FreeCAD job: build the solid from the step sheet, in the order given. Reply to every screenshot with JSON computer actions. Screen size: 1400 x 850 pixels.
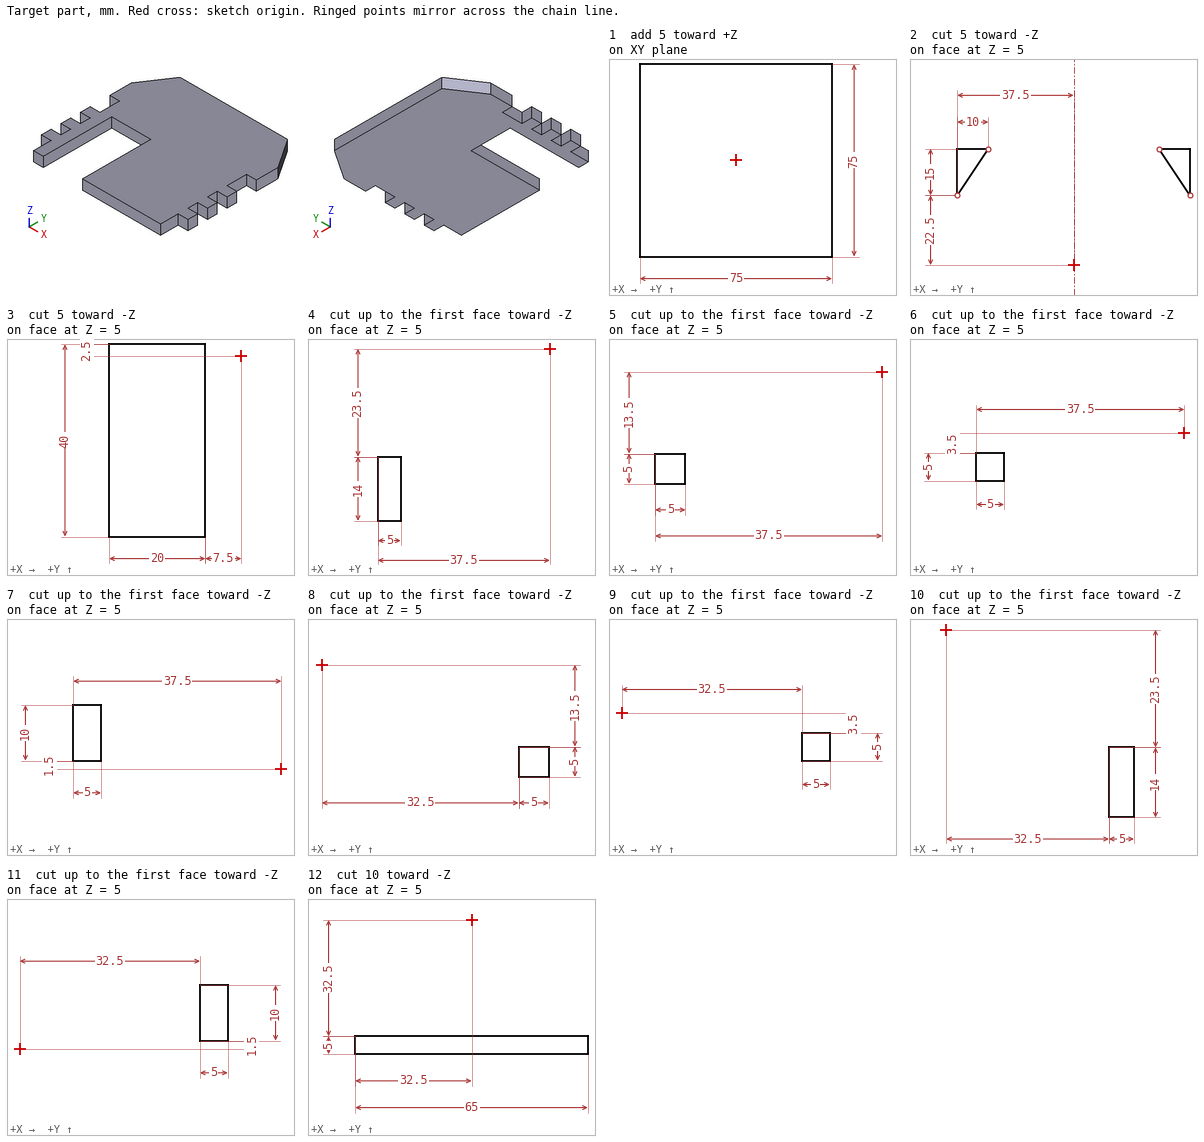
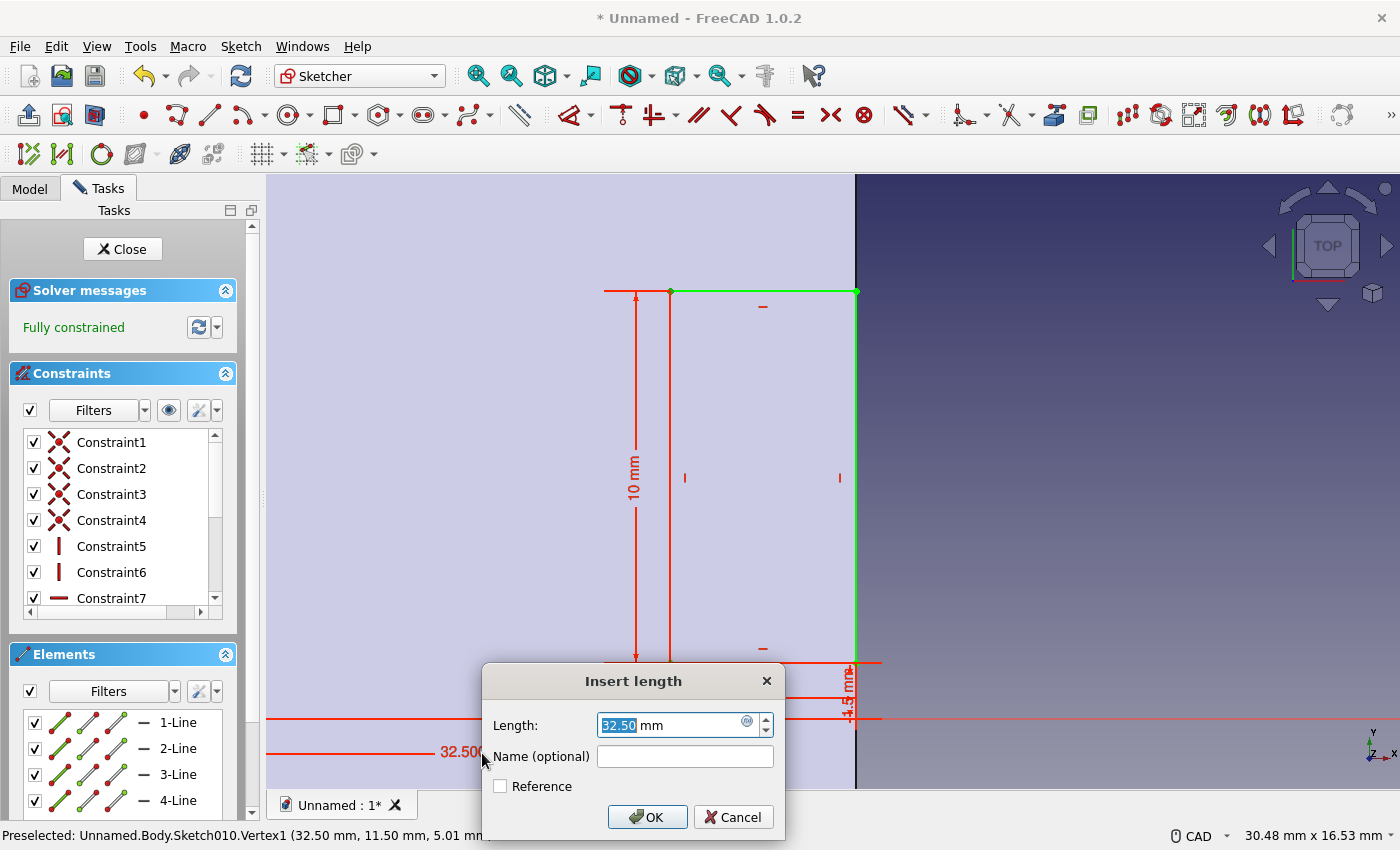
{"action": "type", "text": "32.5"}
{"action": "key", "text": "Return"}
{"action": "key", "text": "Escape"}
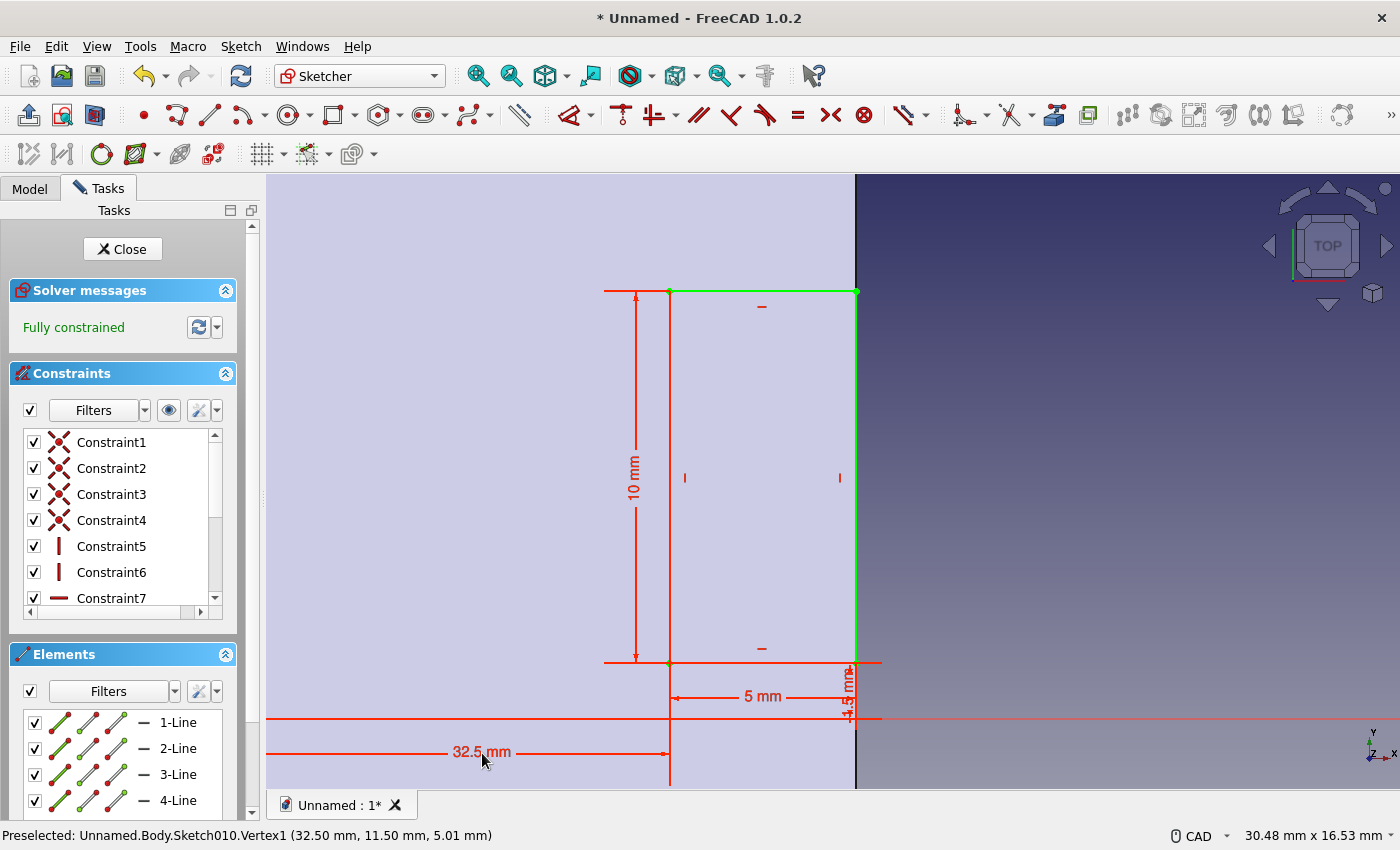
{"action": "left_click", "coordinate": [123, 249]}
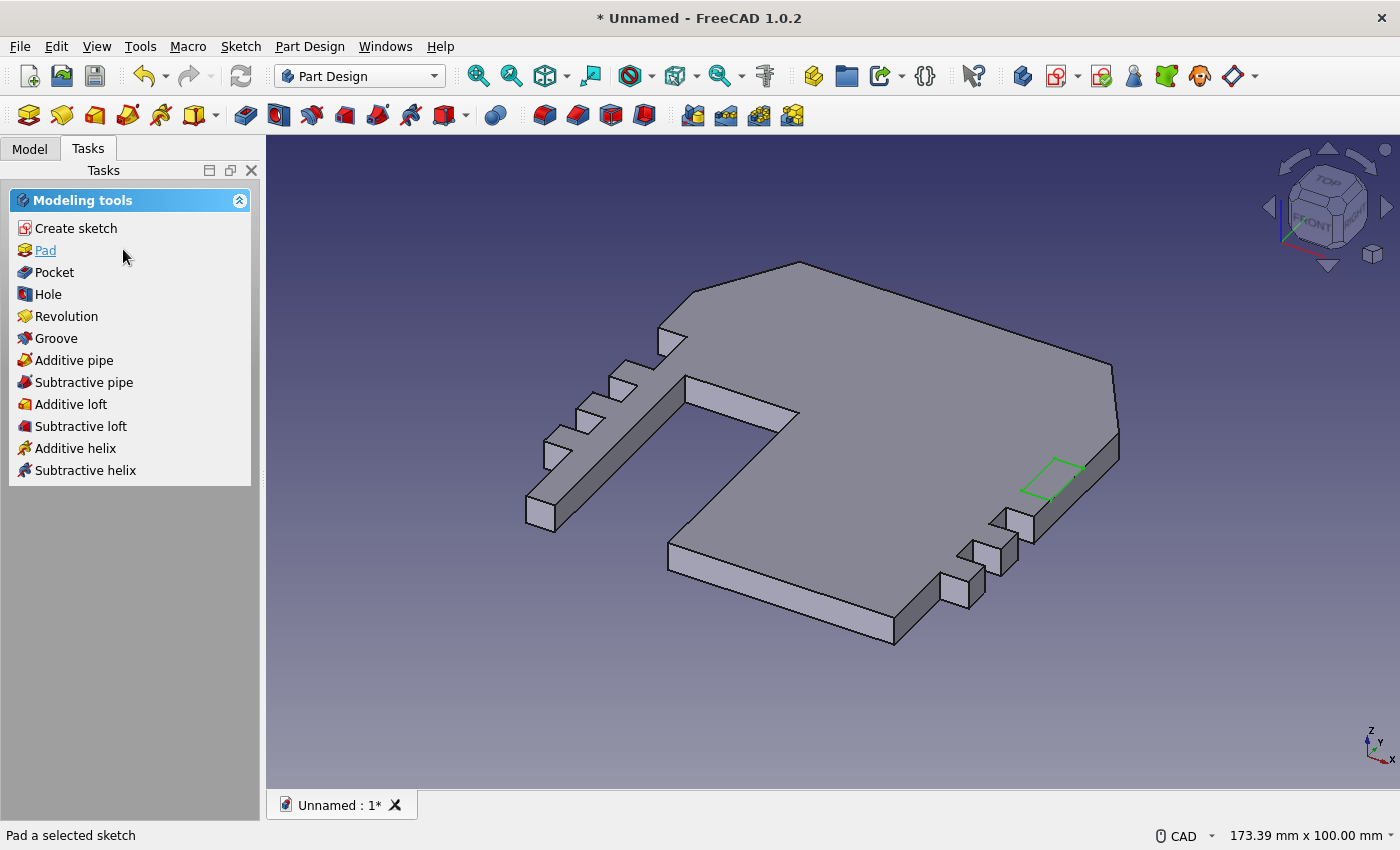
{"action": "left_click", "coordinate": [246, 116]}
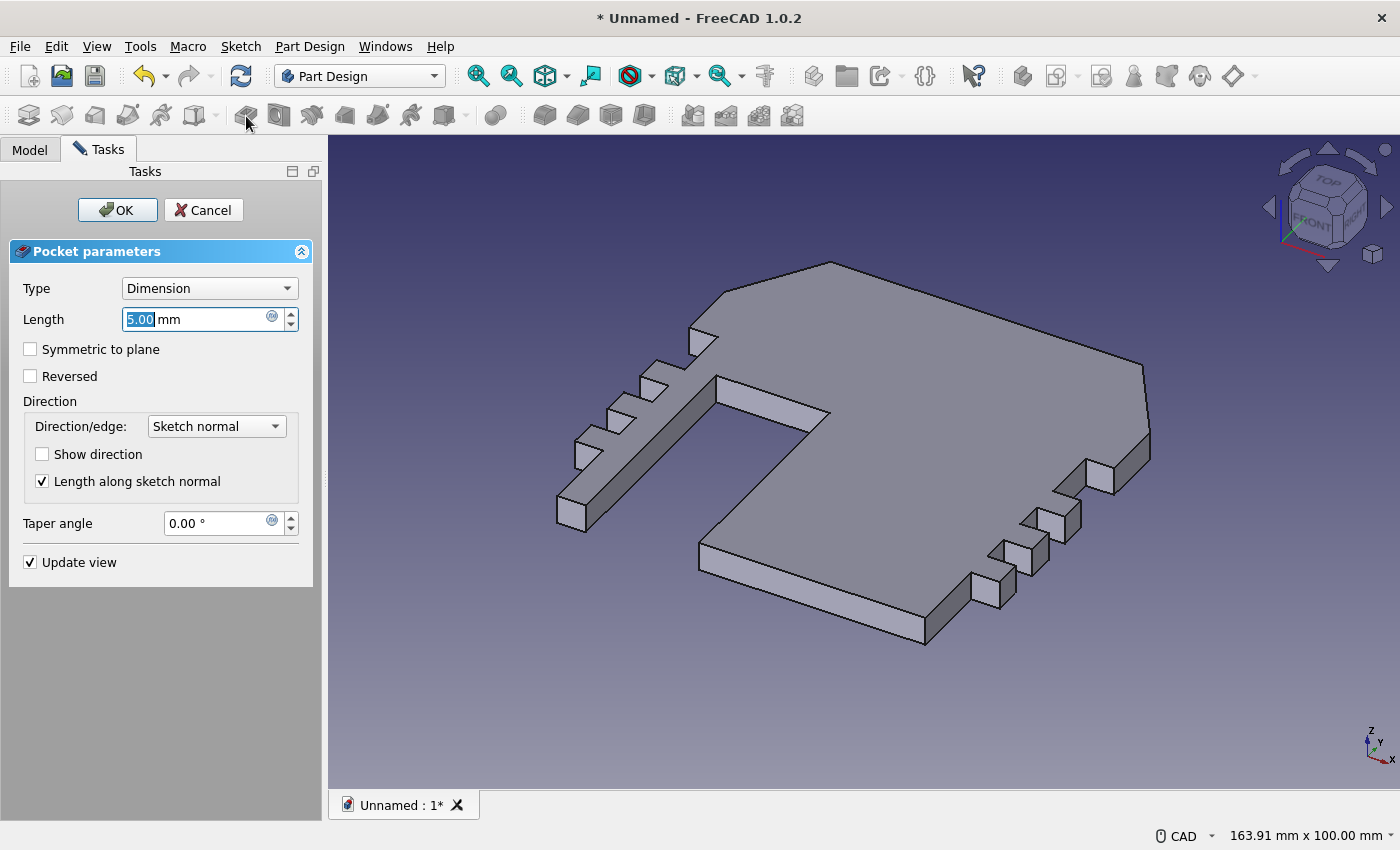
{"action": "left_click", "coordinate": [210, 288]}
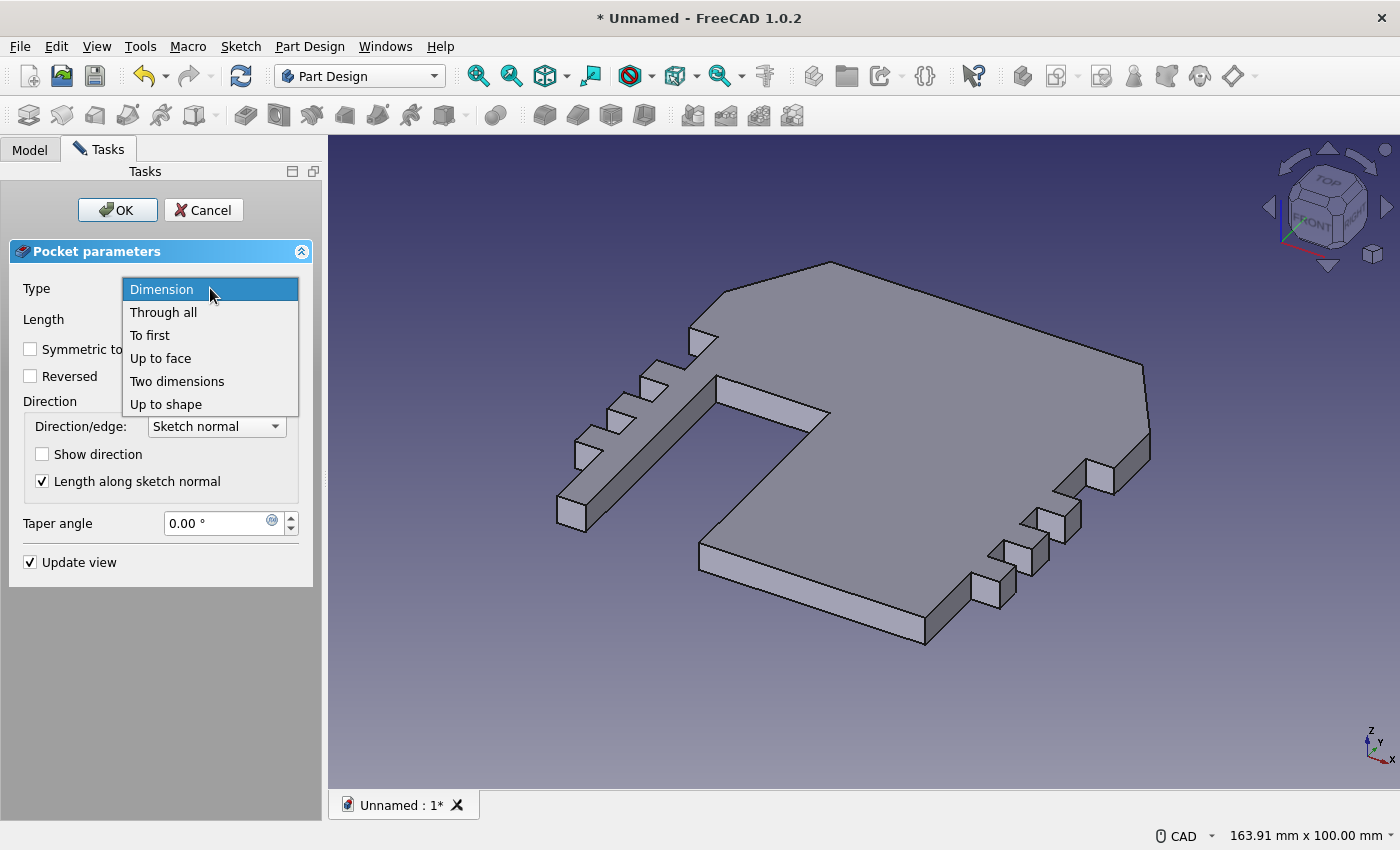
{"action": "left_click", "coordinate": [208, 336]}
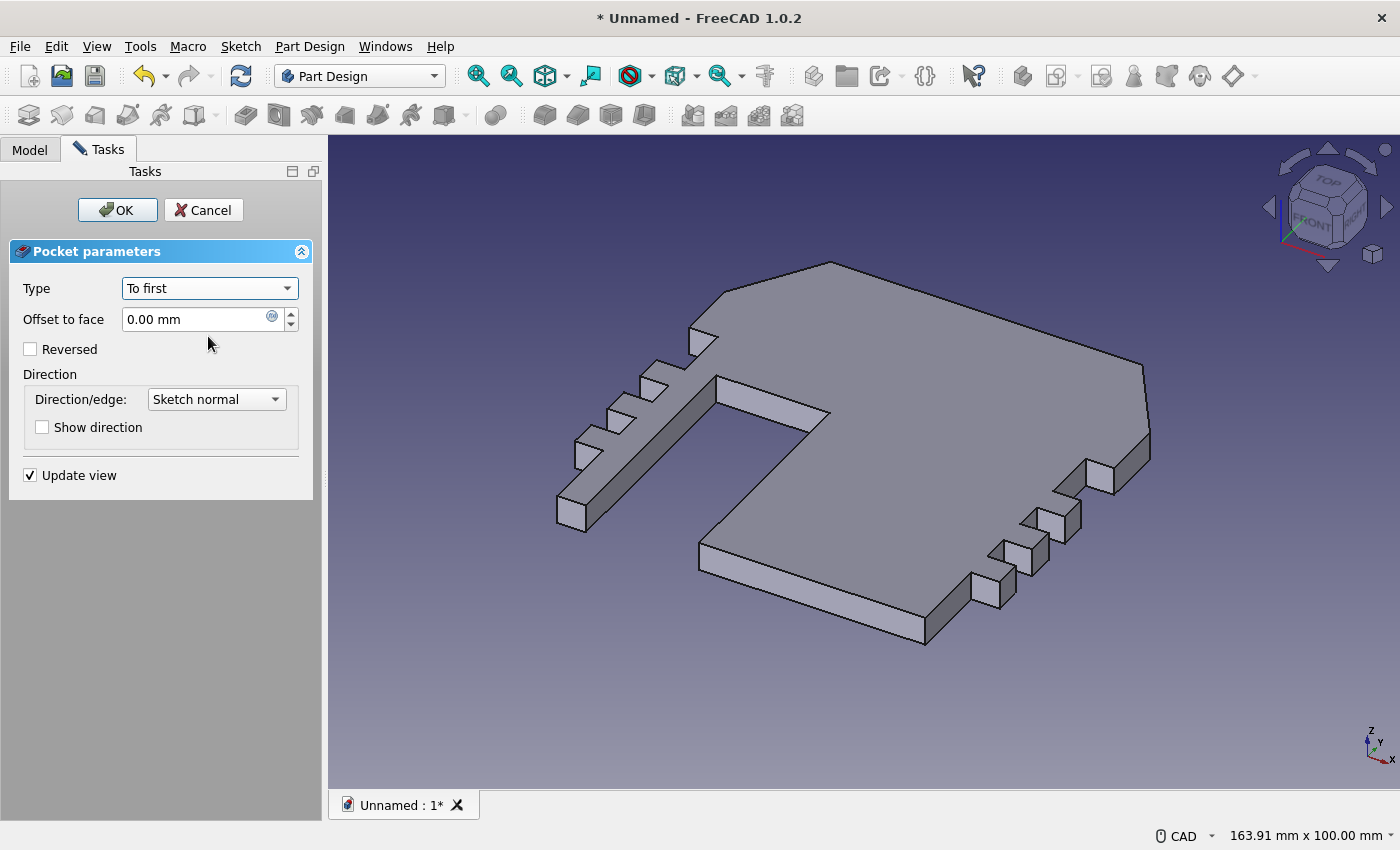
{"action": "left_click", "coordinate": [118, 210]}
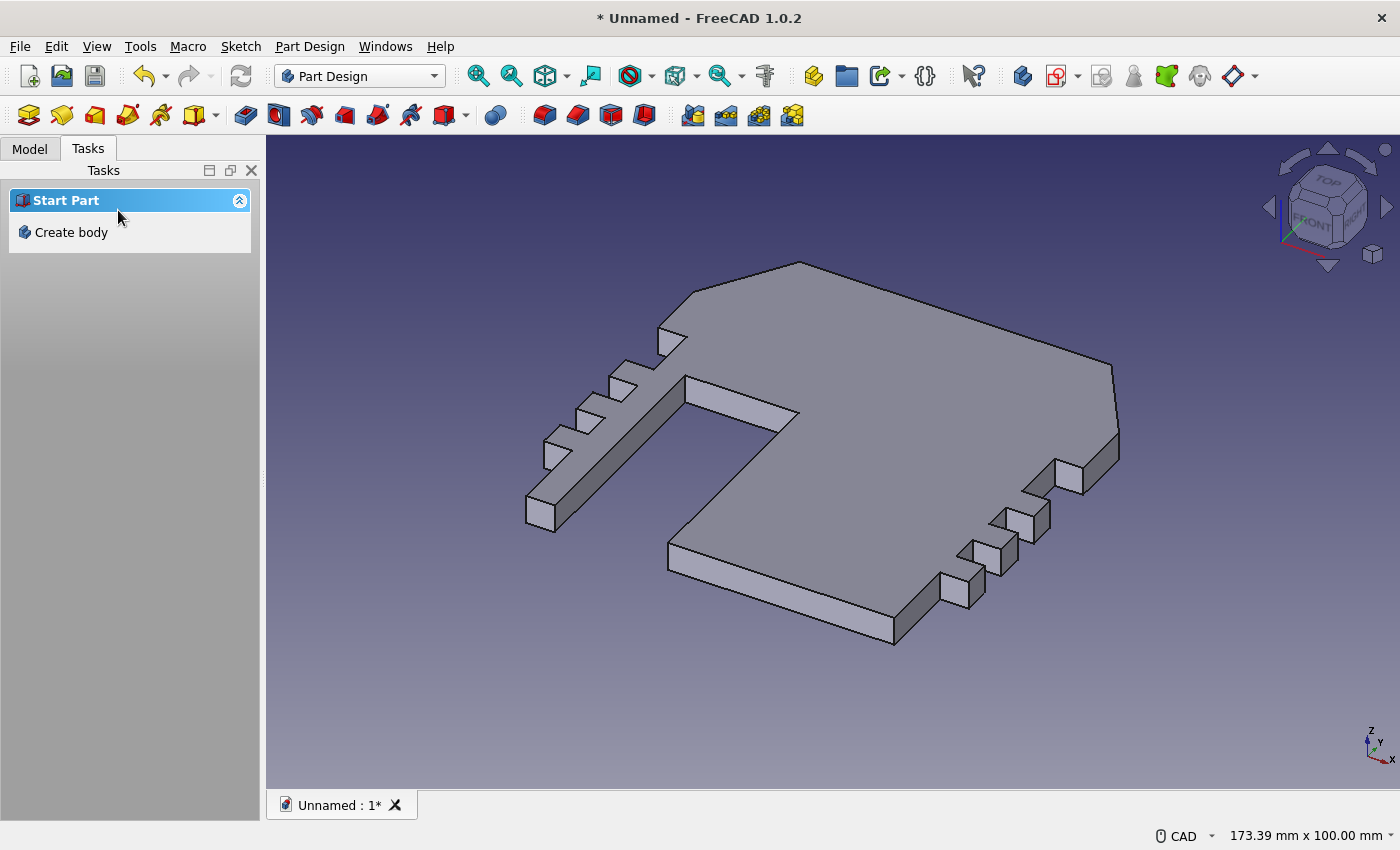
{"action": "left_click", "coordinate": [929, 420]}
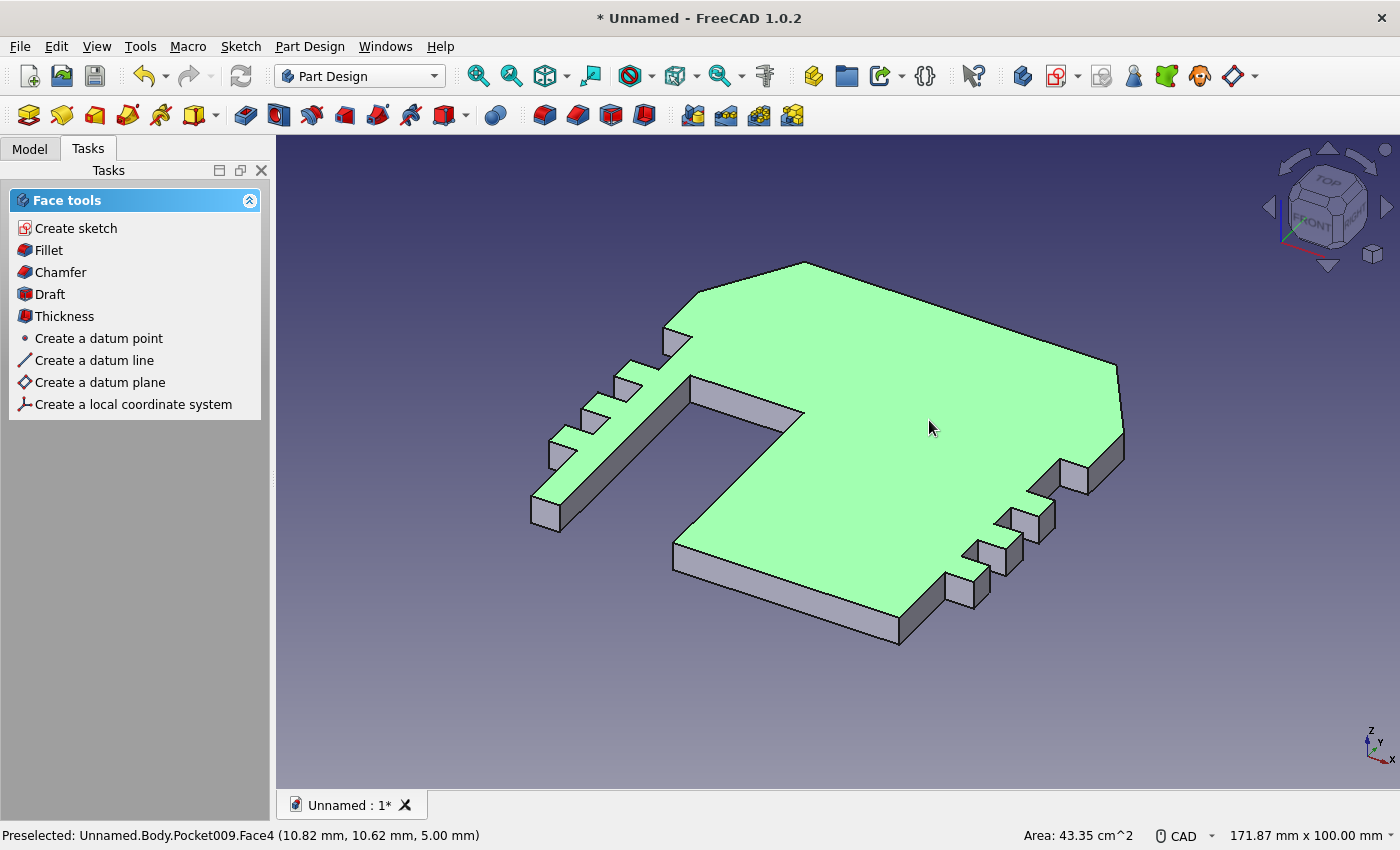
{"action": "left_click", "coordinate": [1056, 76]}